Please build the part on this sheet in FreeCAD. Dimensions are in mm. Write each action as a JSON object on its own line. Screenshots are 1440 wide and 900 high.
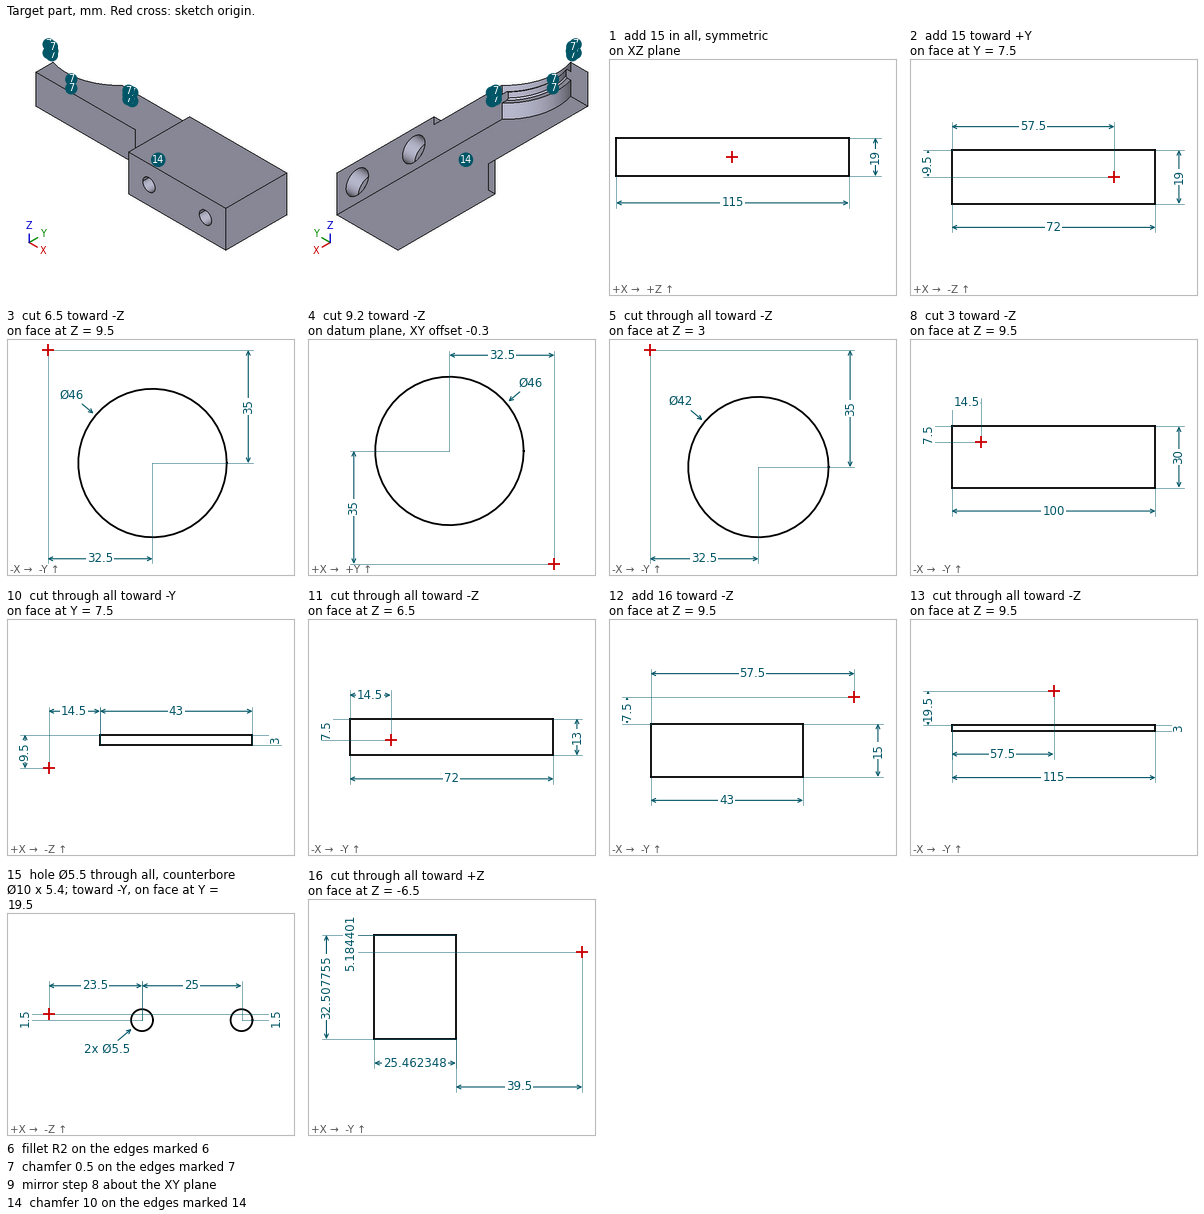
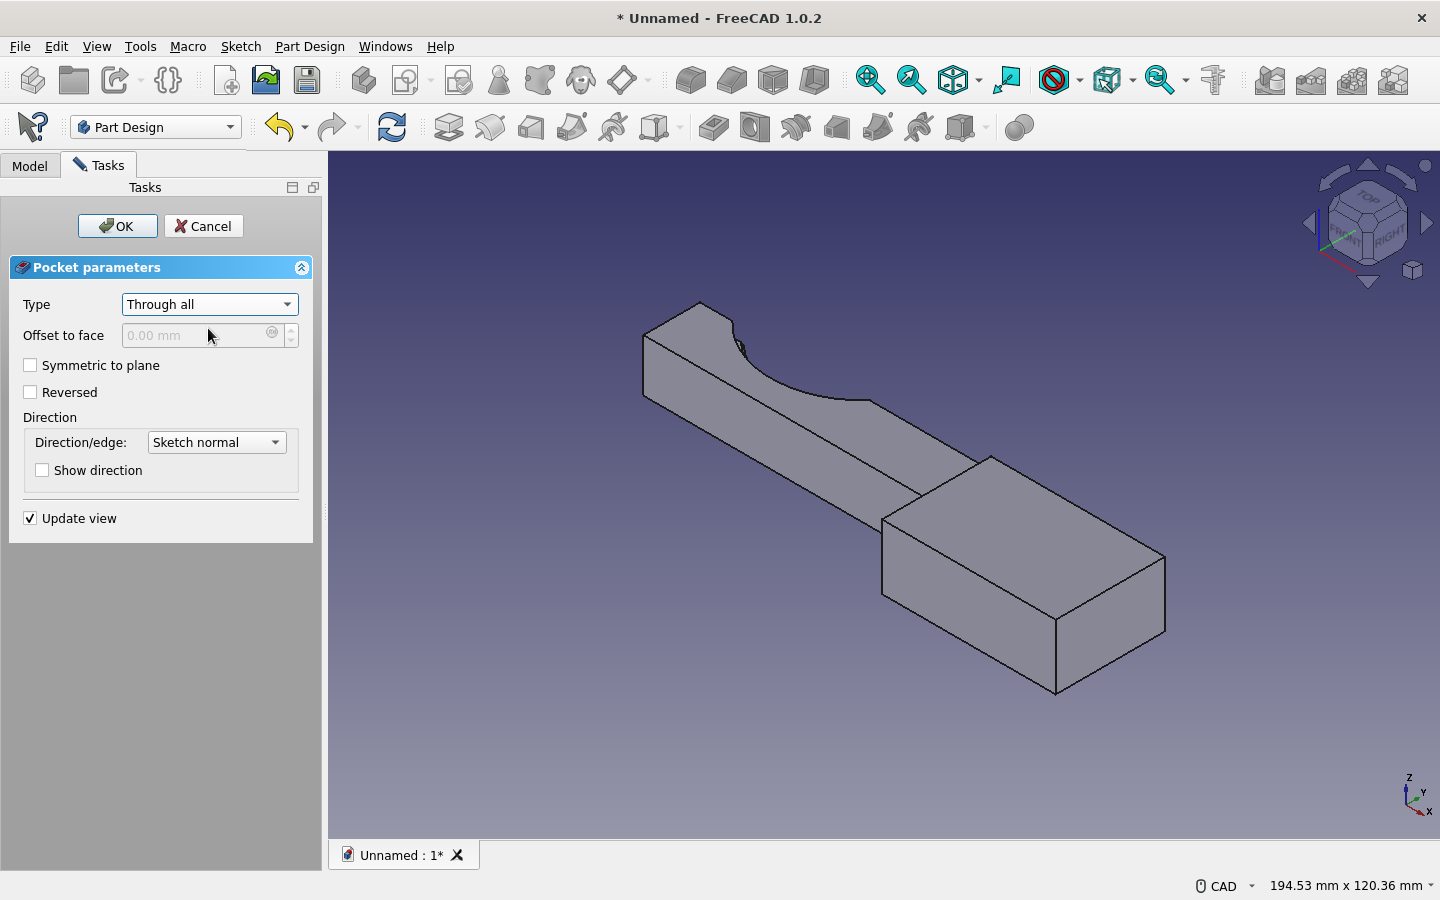
{"action": "left_click", "coordinate": [118, 226]}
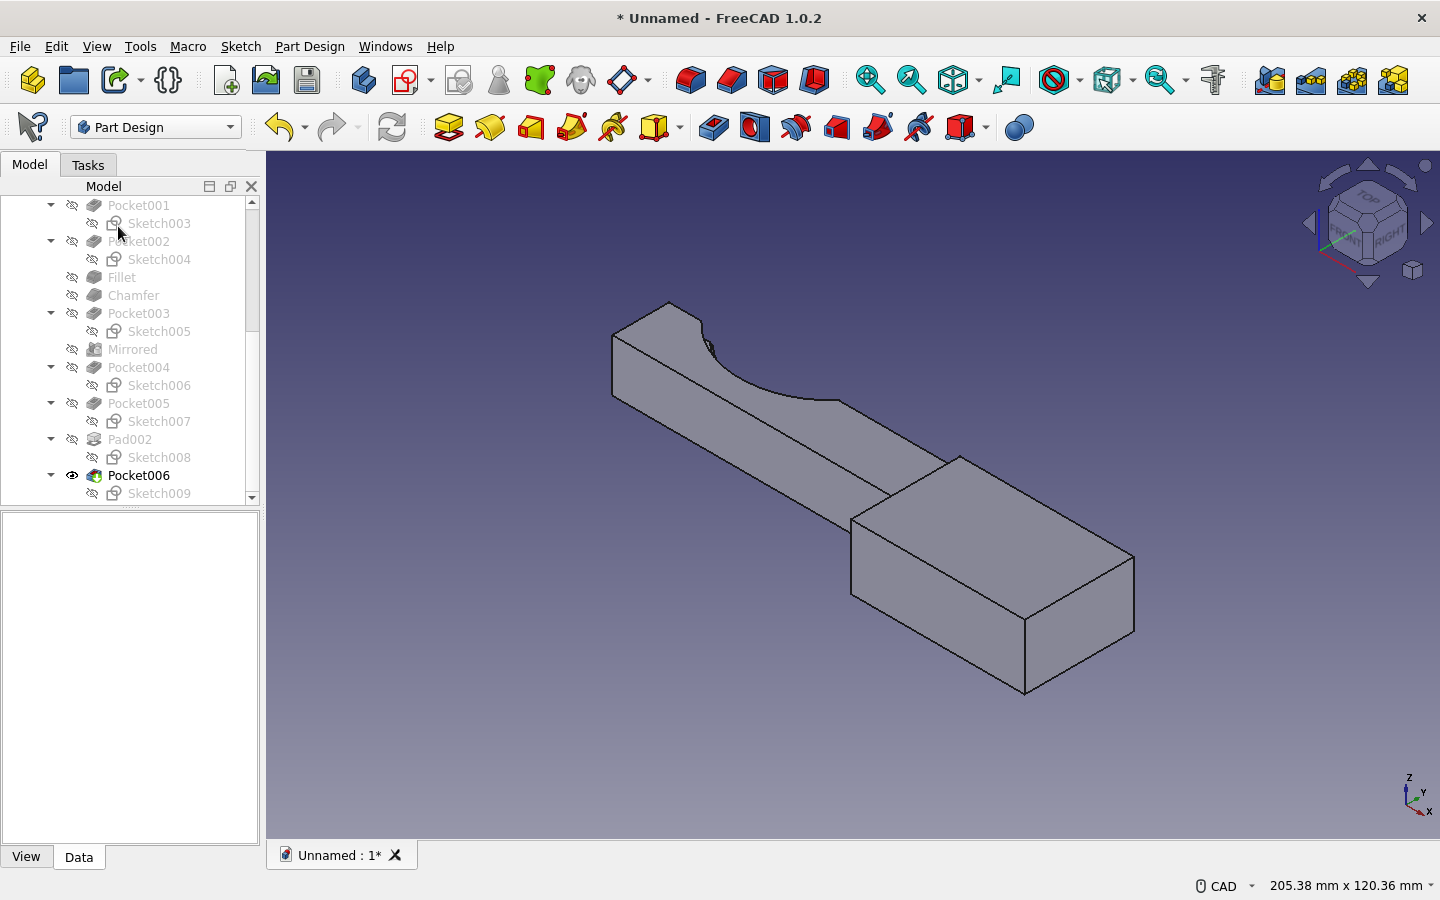
{"action": "key", "text": "2"}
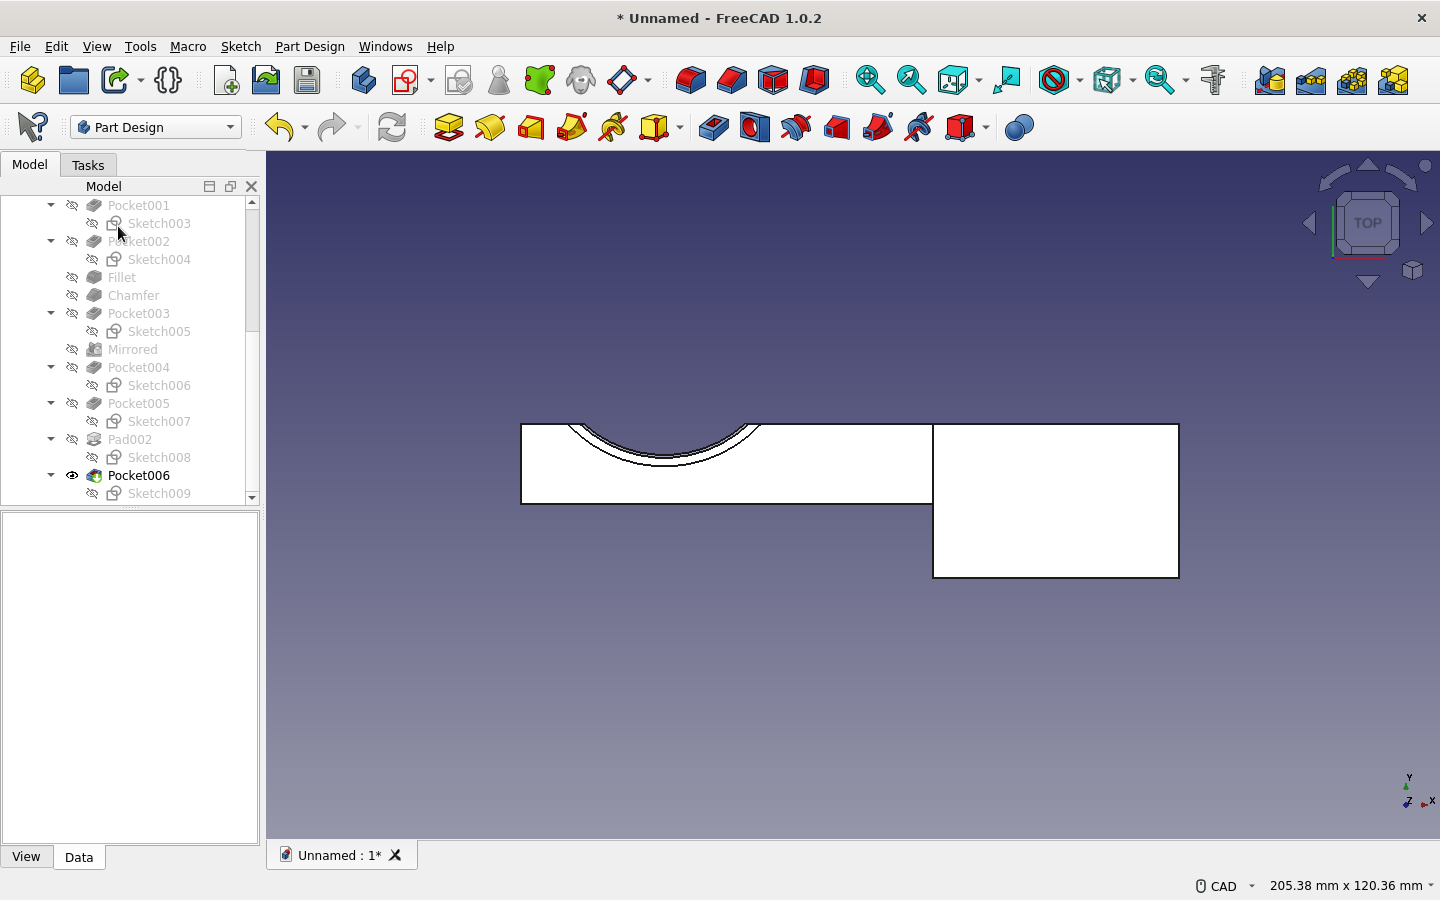
{"action": "key", "text": "0"}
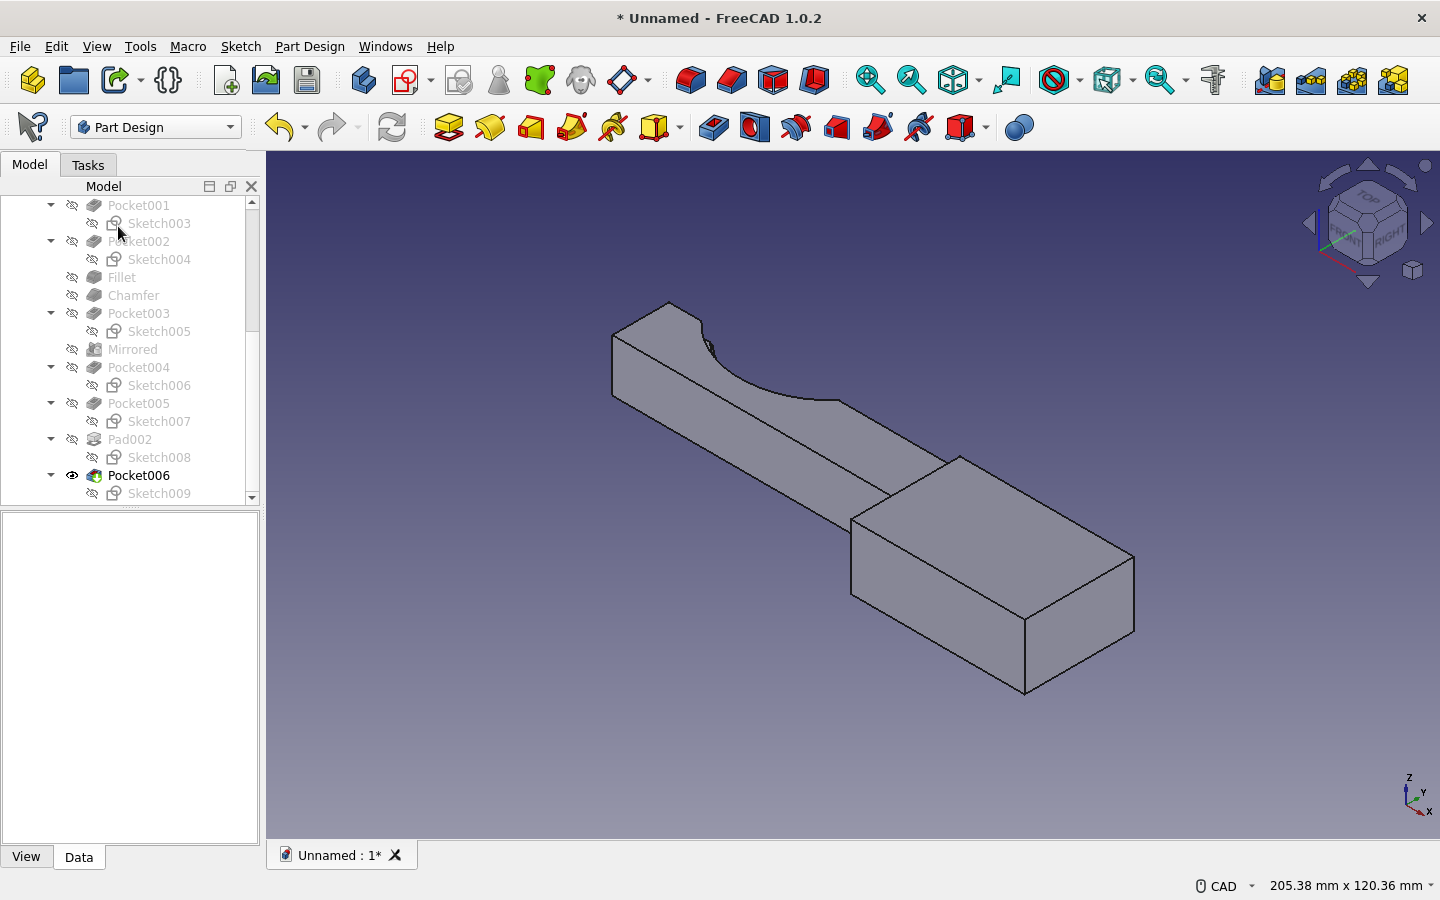
{"action": "key", "text": "1"}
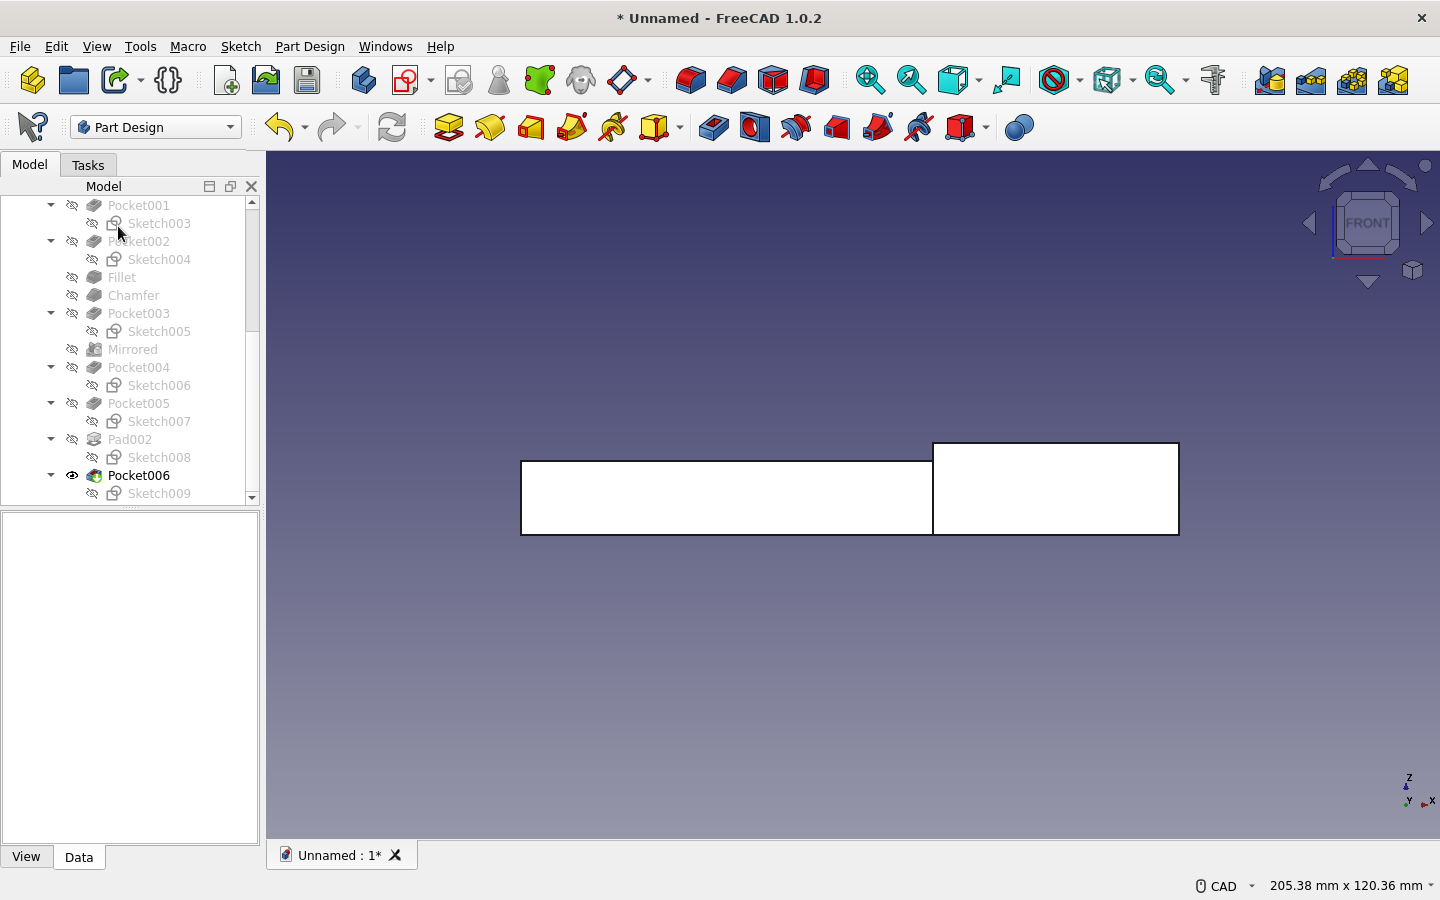
{"action": "key", "text": "3"}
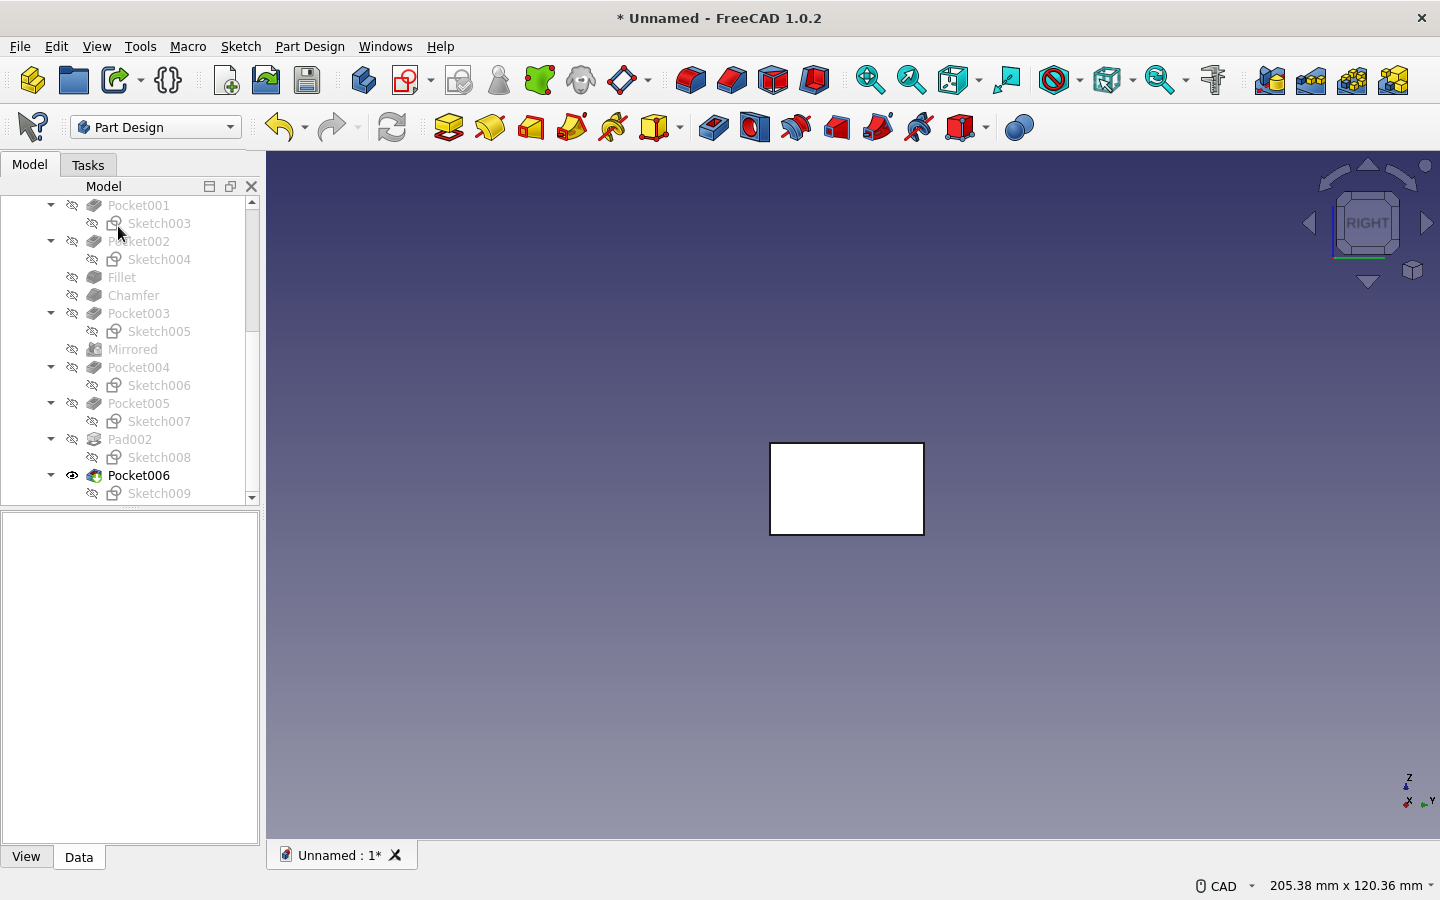
{"action": "left_click", "coordinate": [871, 80]}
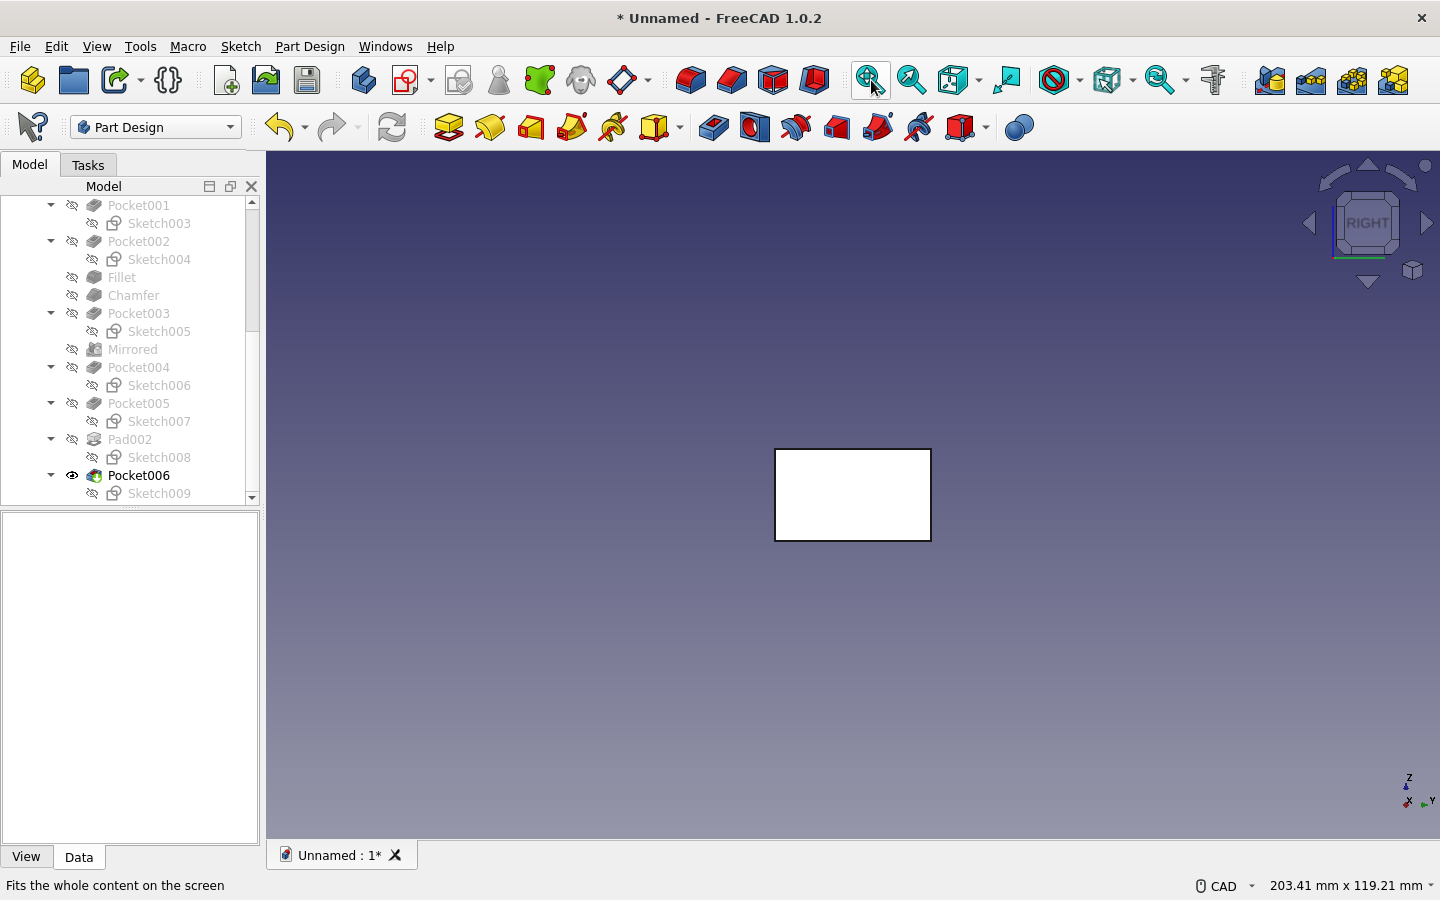
{"action": "key", "text": "5"}